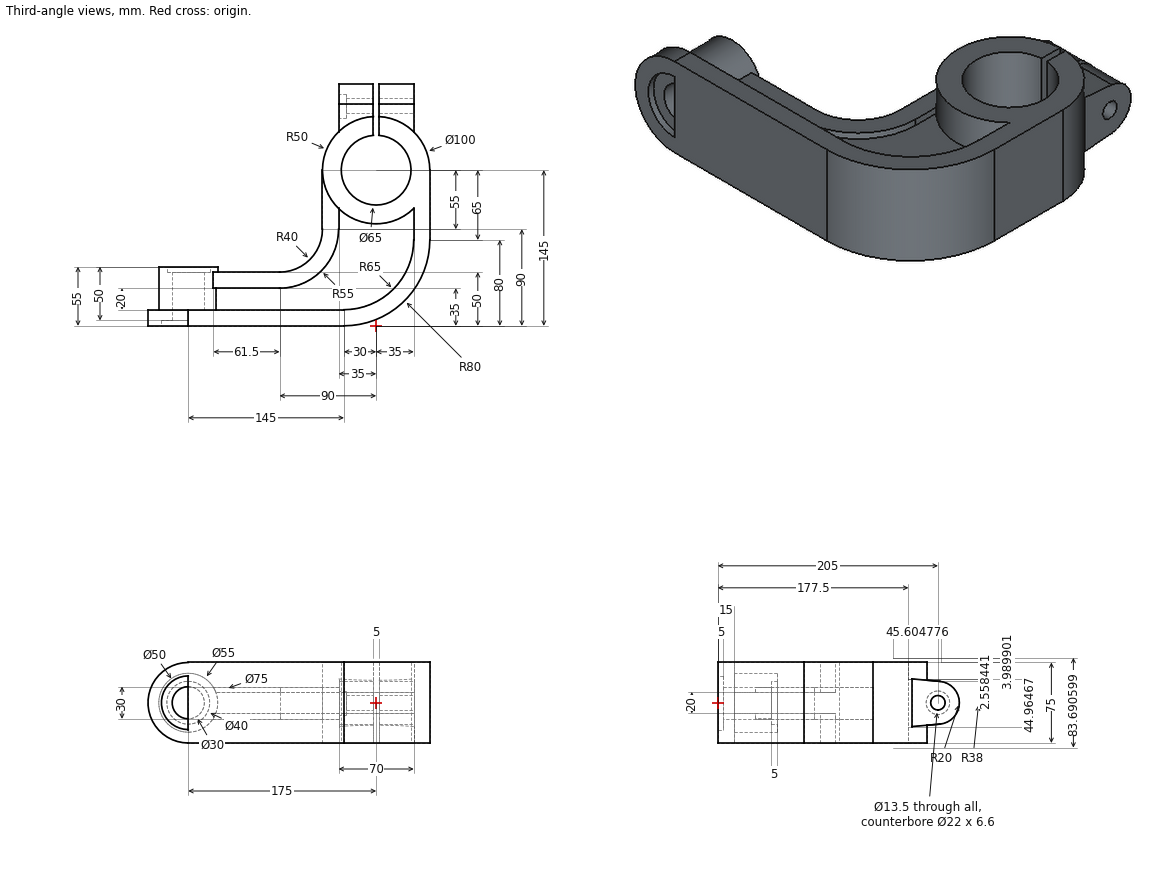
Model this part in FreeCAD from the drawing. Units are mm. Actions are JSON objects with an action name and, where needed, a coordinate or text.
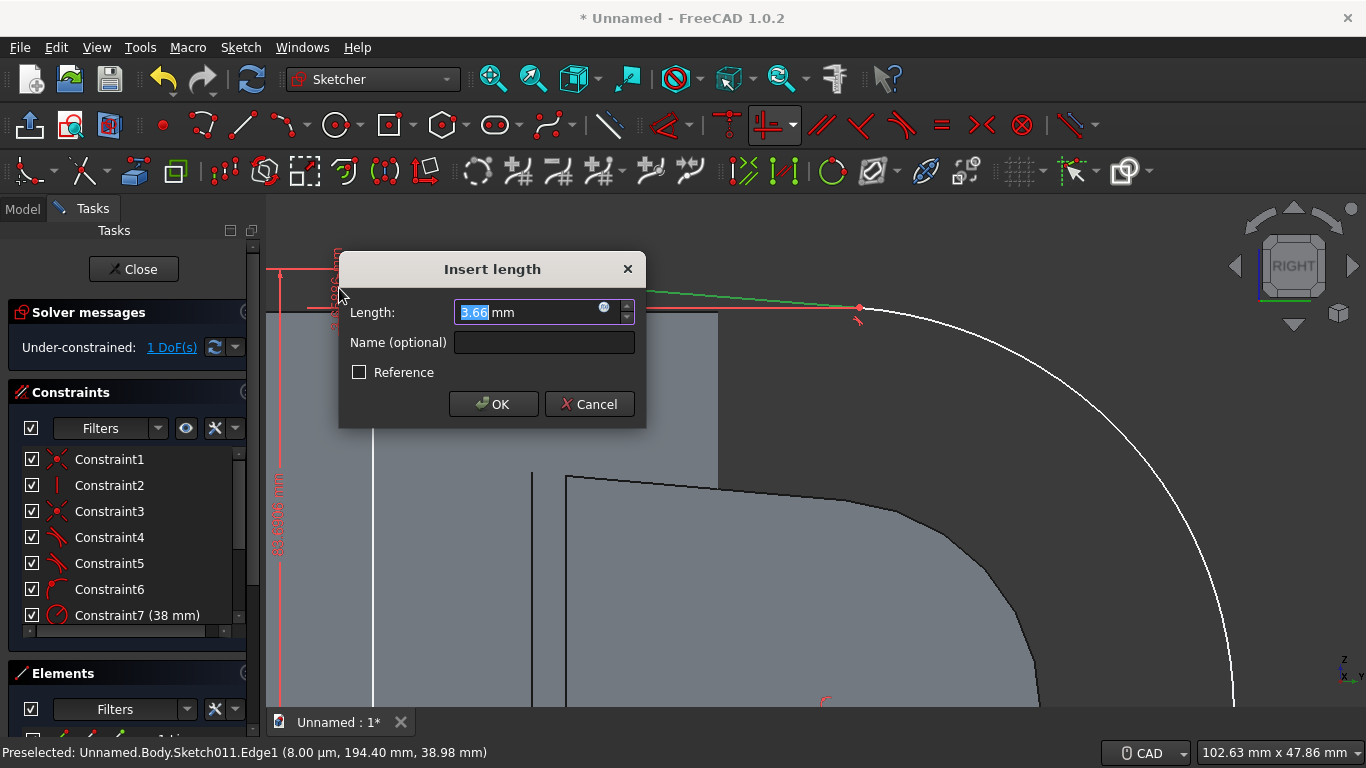
{"action": "type", "text": "3.989901"}
{"action": "key", "text": "Return"}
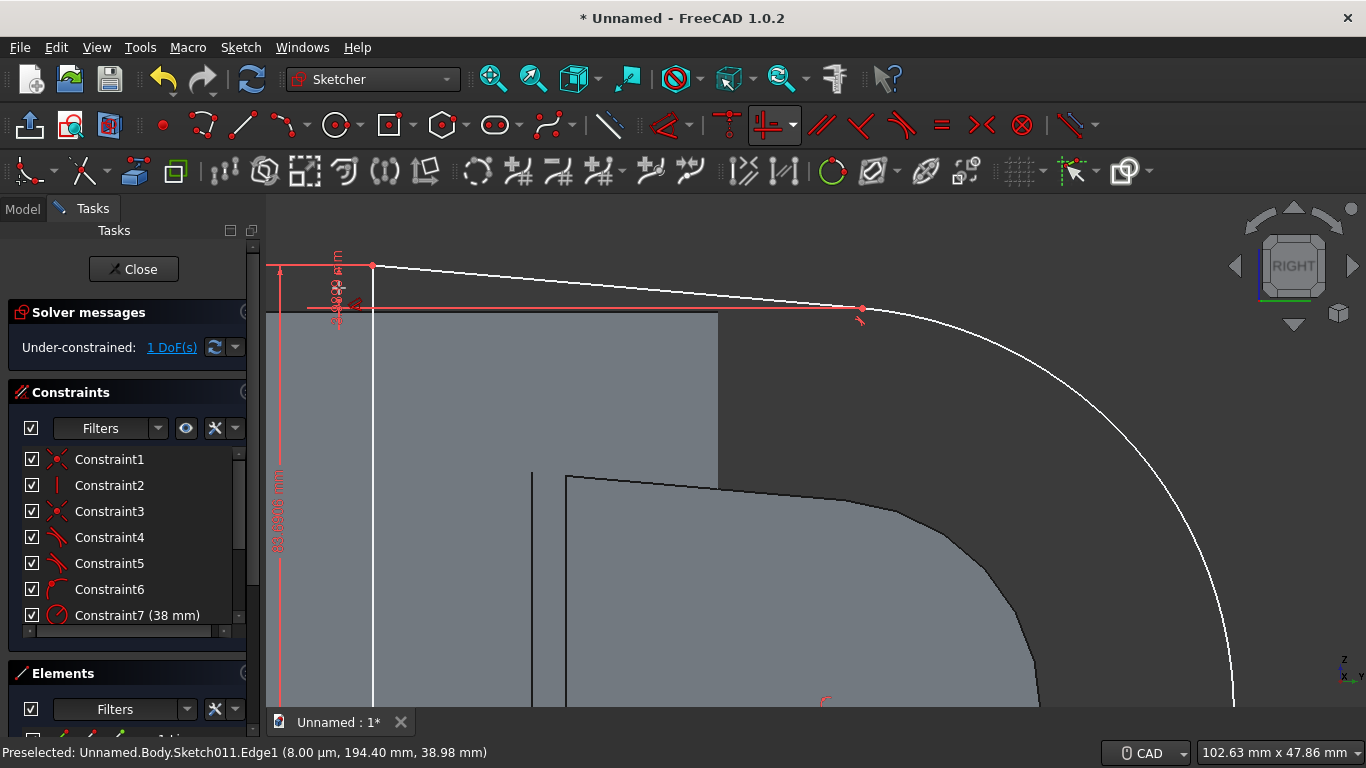
{"action": "left_click", "coordinate": [715, 295]}
{"action": "left_click", "coordinate": [617, 231]}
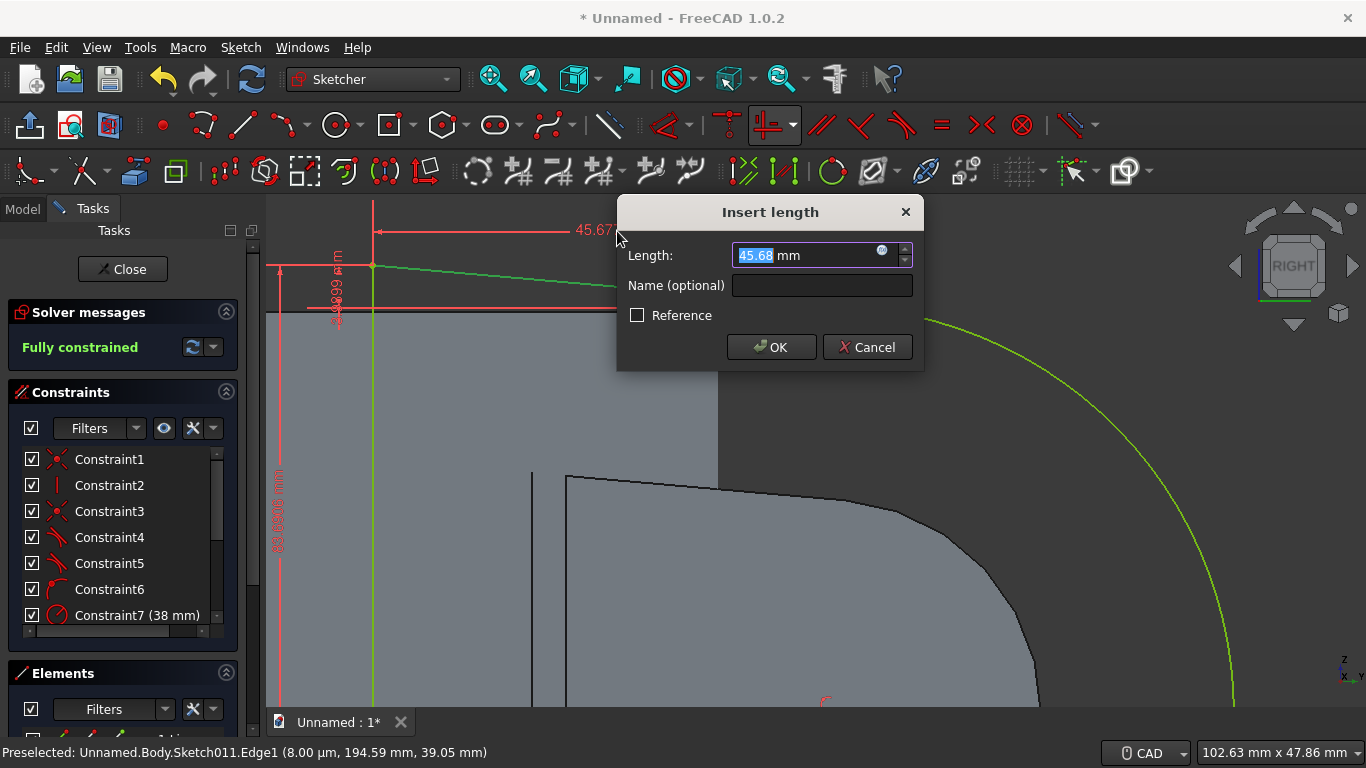
{"action": "type", "text": "45.604776"}
{"action": "key", "text": "Return"}
{"action": "key", "text": "Escape"}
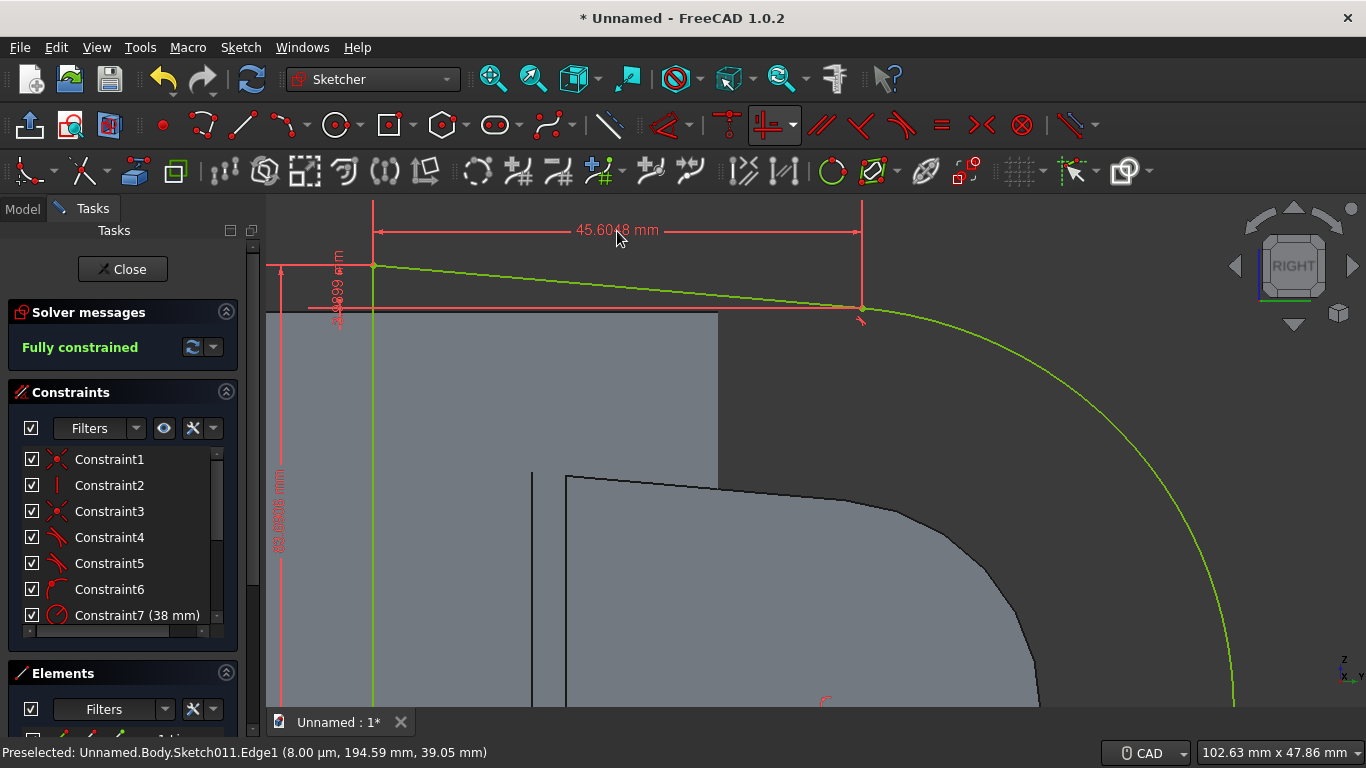
{"action": "left_click", "coordinate": [123, 269]}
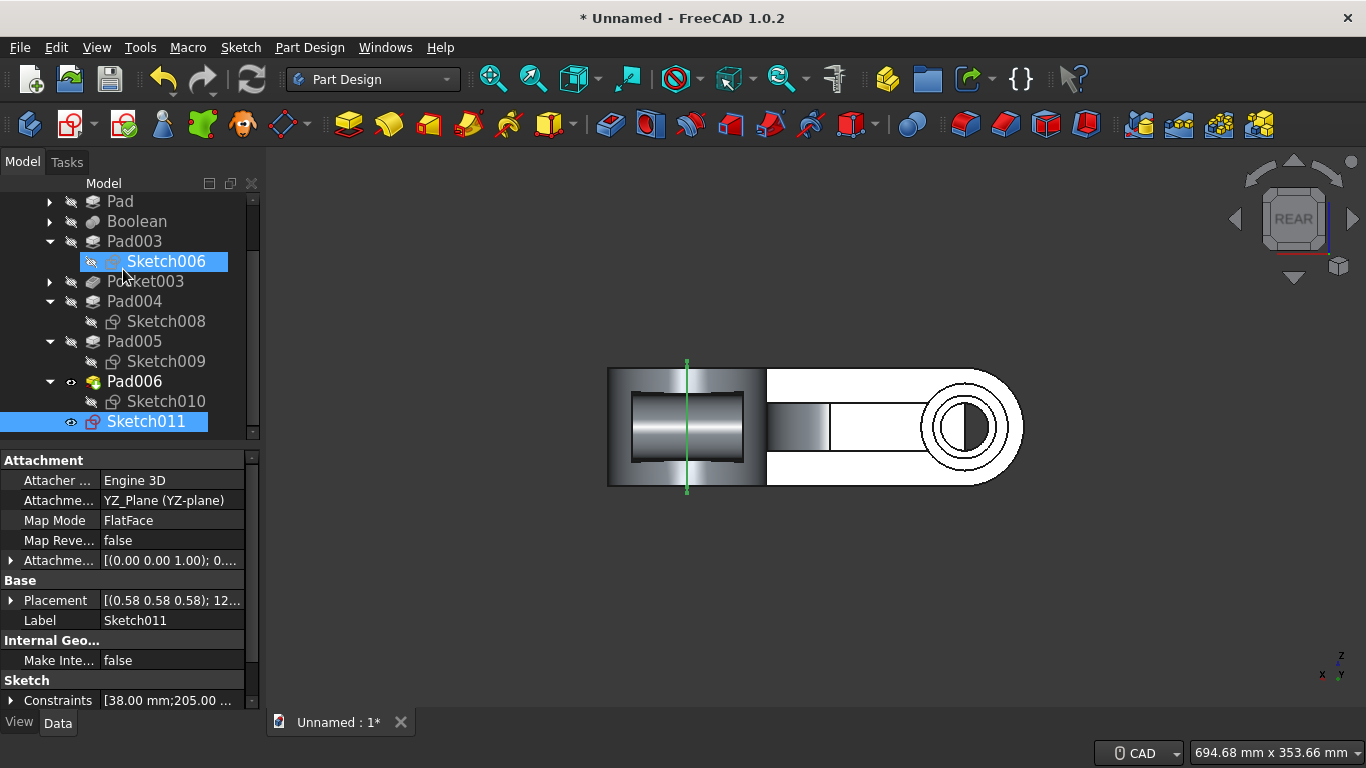
{"action": "left_click", "coordinate": [612, 124]}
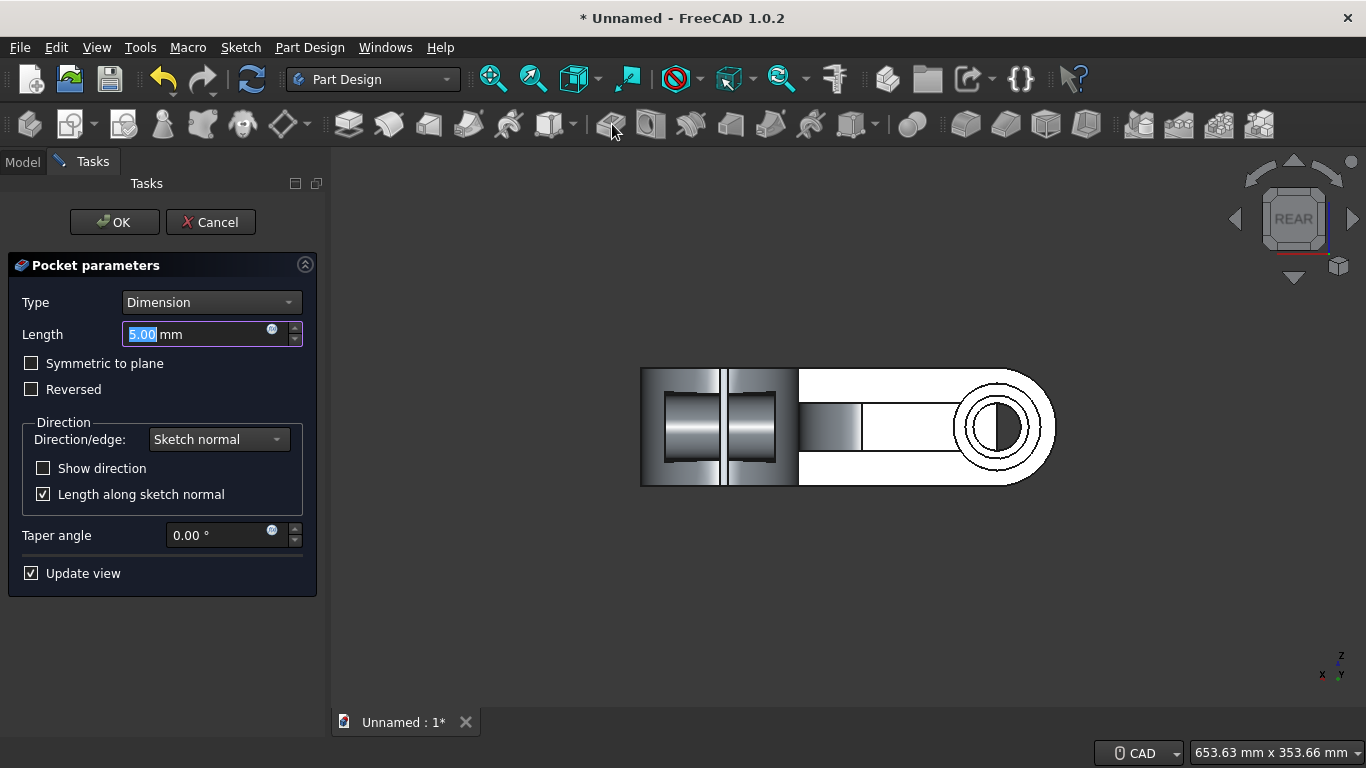
{"action": "type", "text": "5"}
{"action": "key", "text": "Tab"}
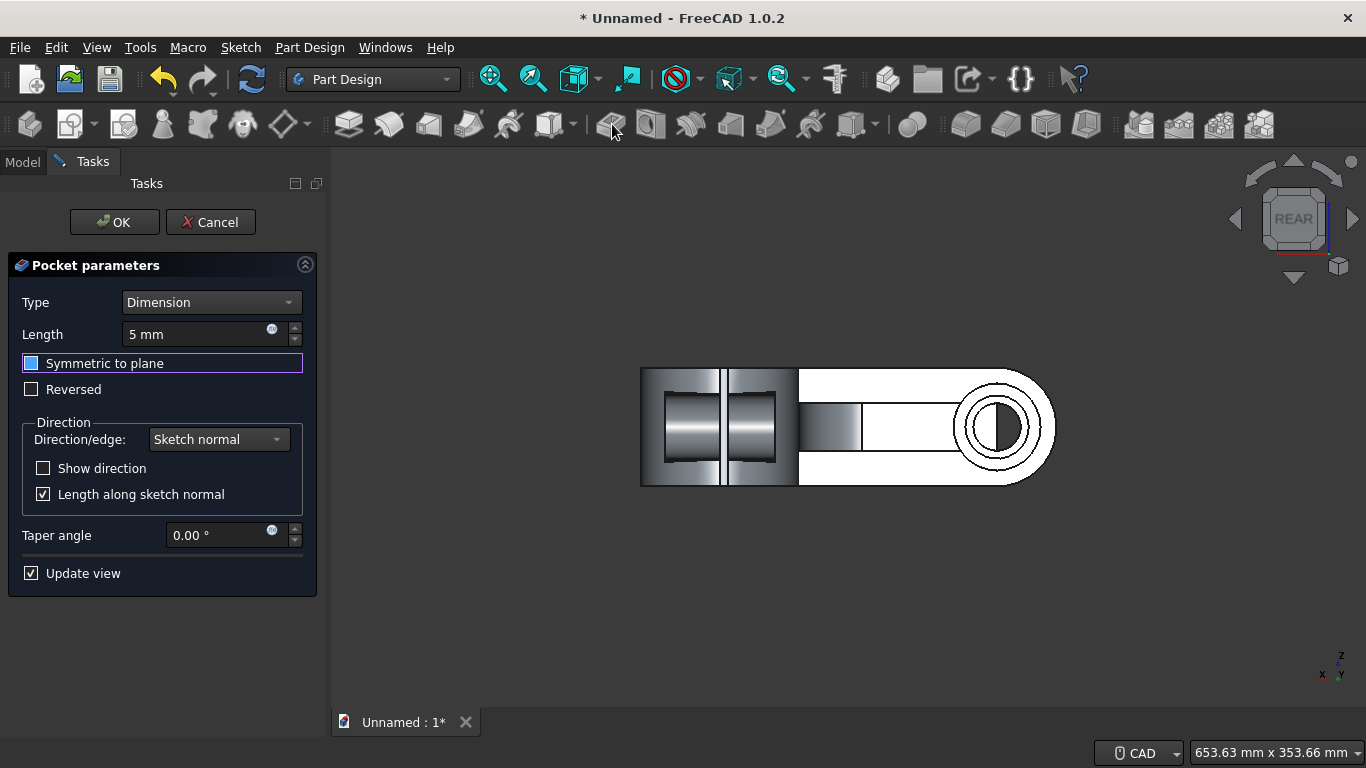
{"action": "left_click", "coordinate": [30, 363]}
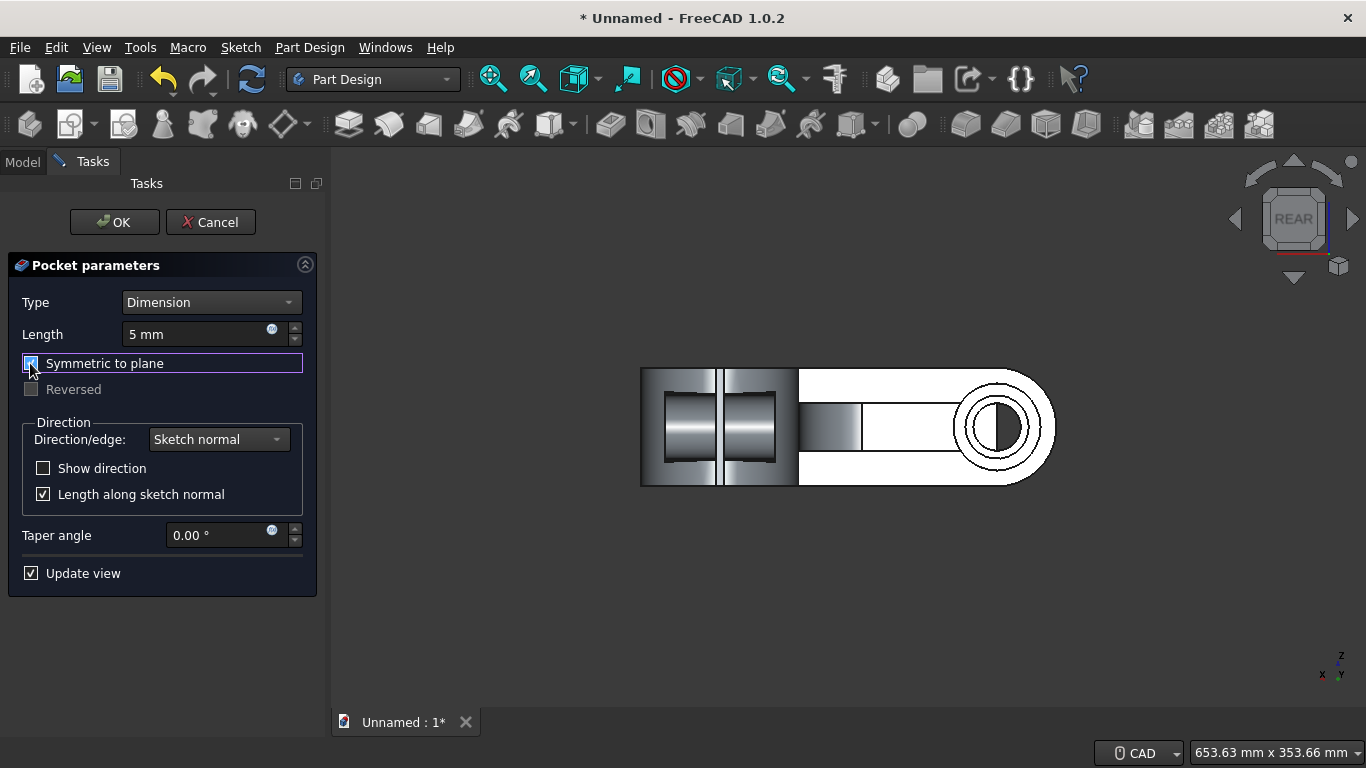
{"action": "left_click", "coordinate": [115, 222]}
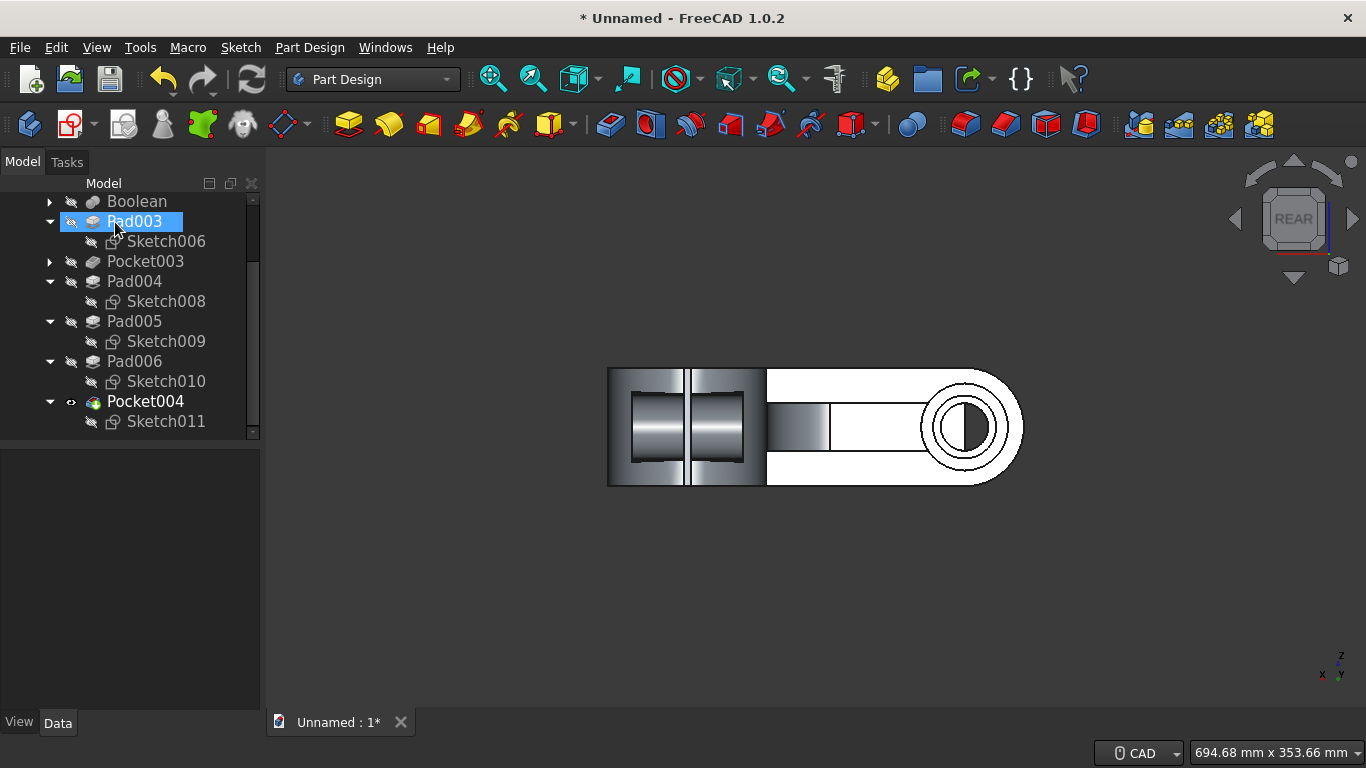
{"action": "left_click", "coordinate": [494, 80]}